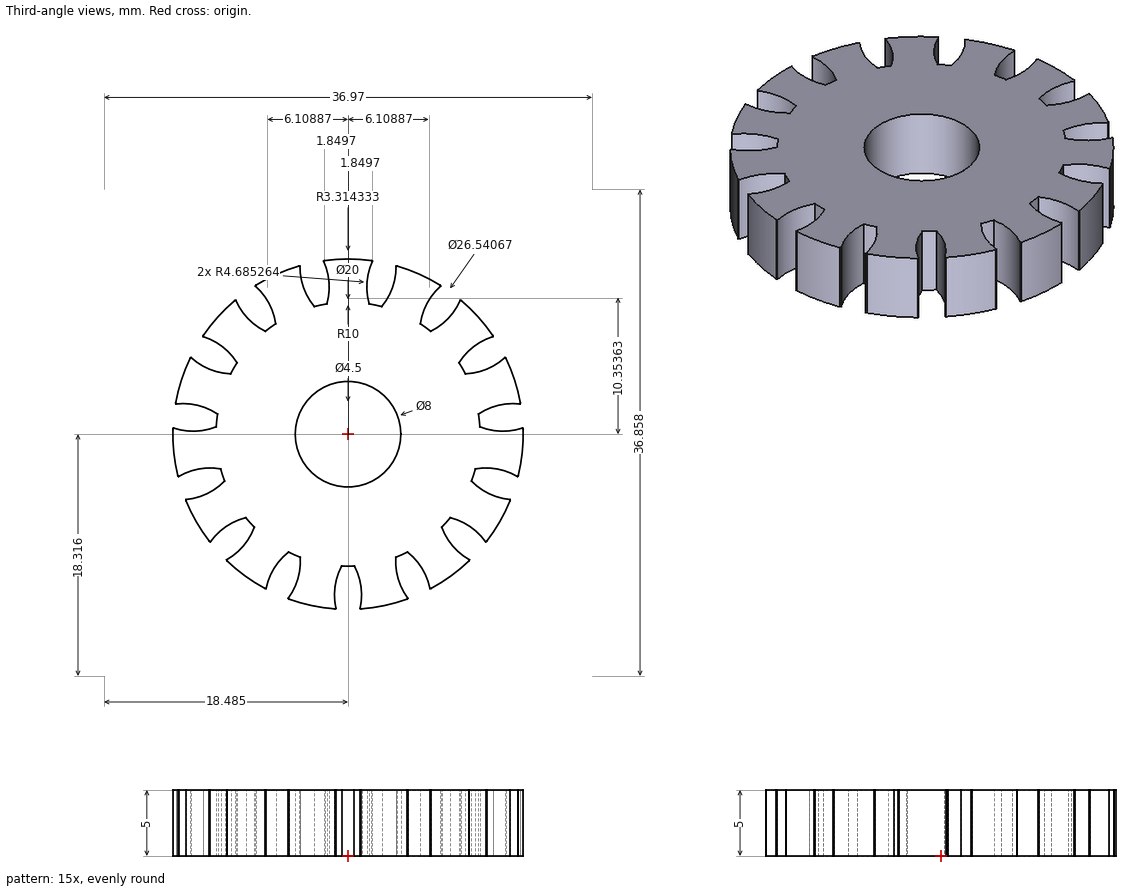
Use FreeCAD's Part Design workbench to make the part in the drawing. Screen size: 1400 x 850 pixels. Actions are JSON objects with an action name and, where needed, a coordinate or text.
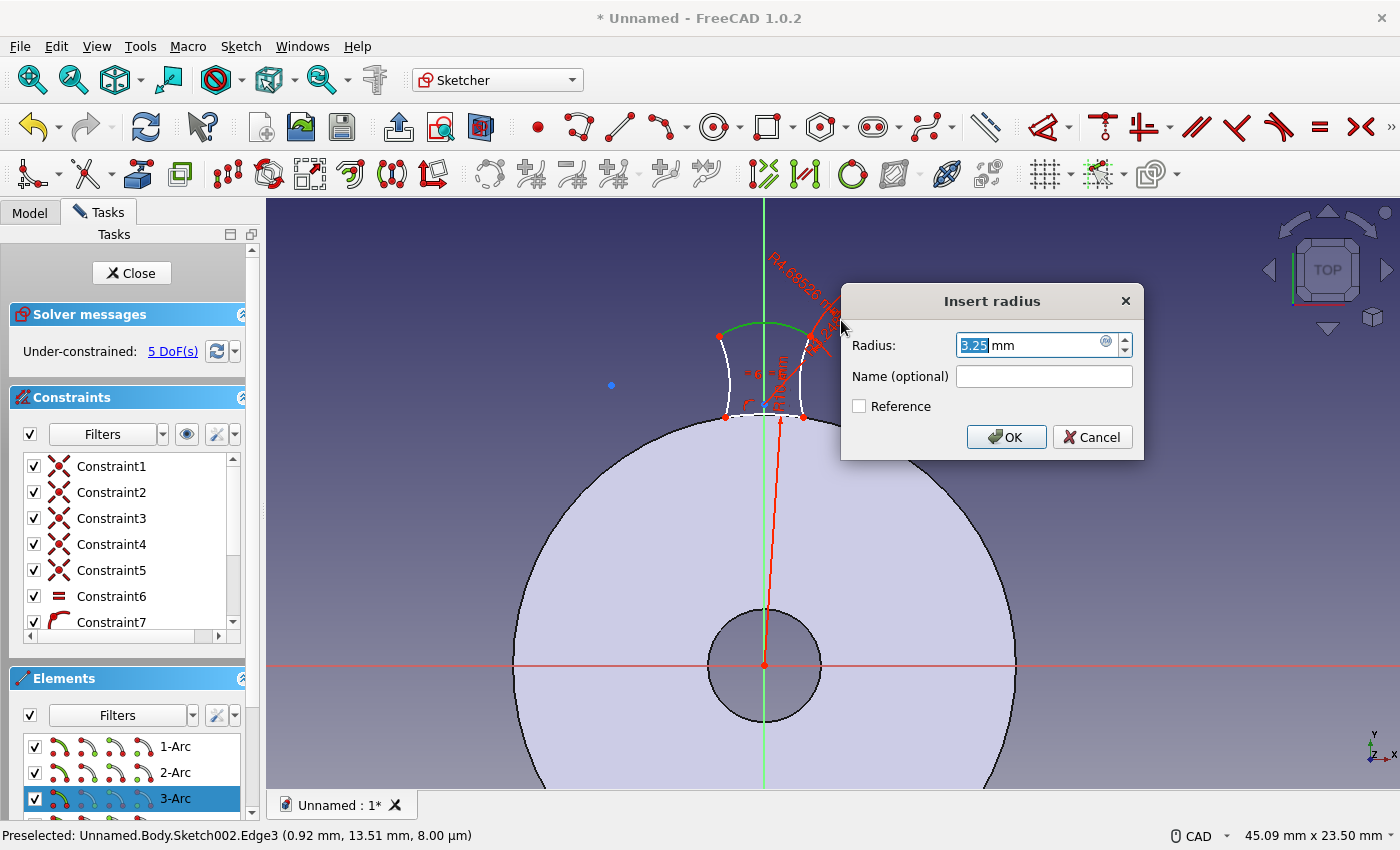
{"action": "type", "text": "3.314333"}
{"action": "key", "text": "Return"}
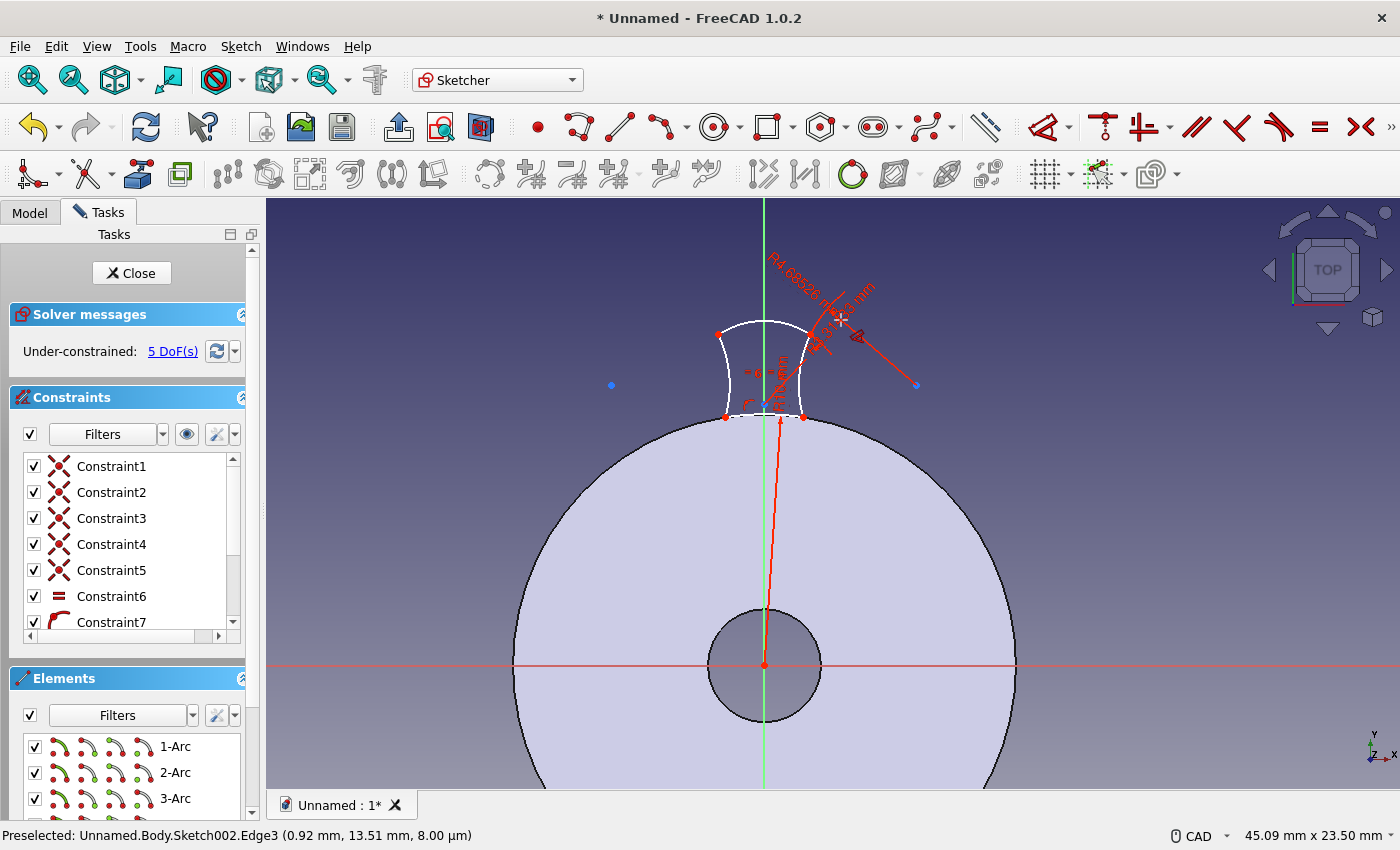
{"action": "left_click", "coordinate": [810, 335]}
{"action": "left_click", "coordinate": [787, 700]}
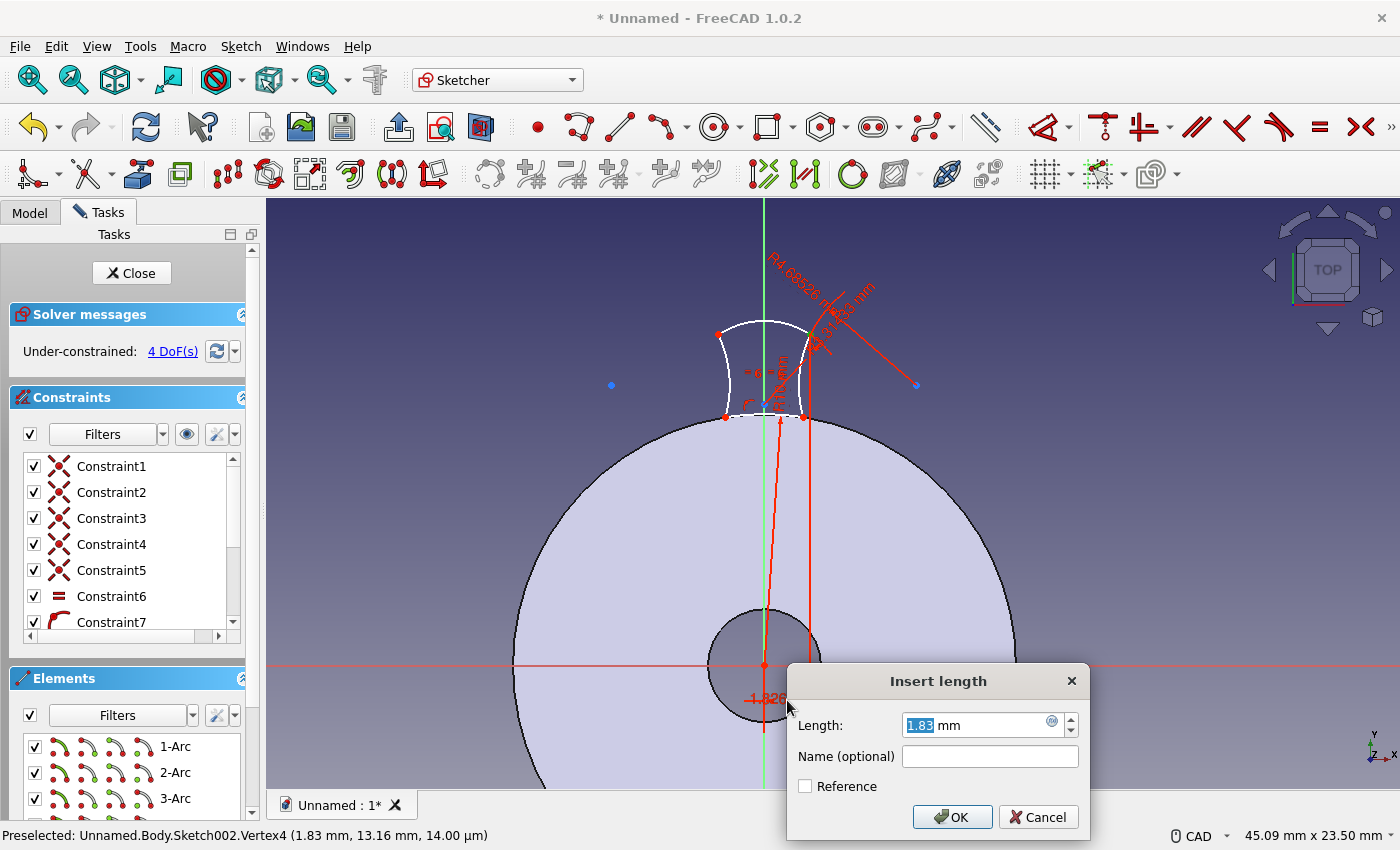
{"action": "type", "text": "1.8497"}
{"action": "key", "text": "Return"}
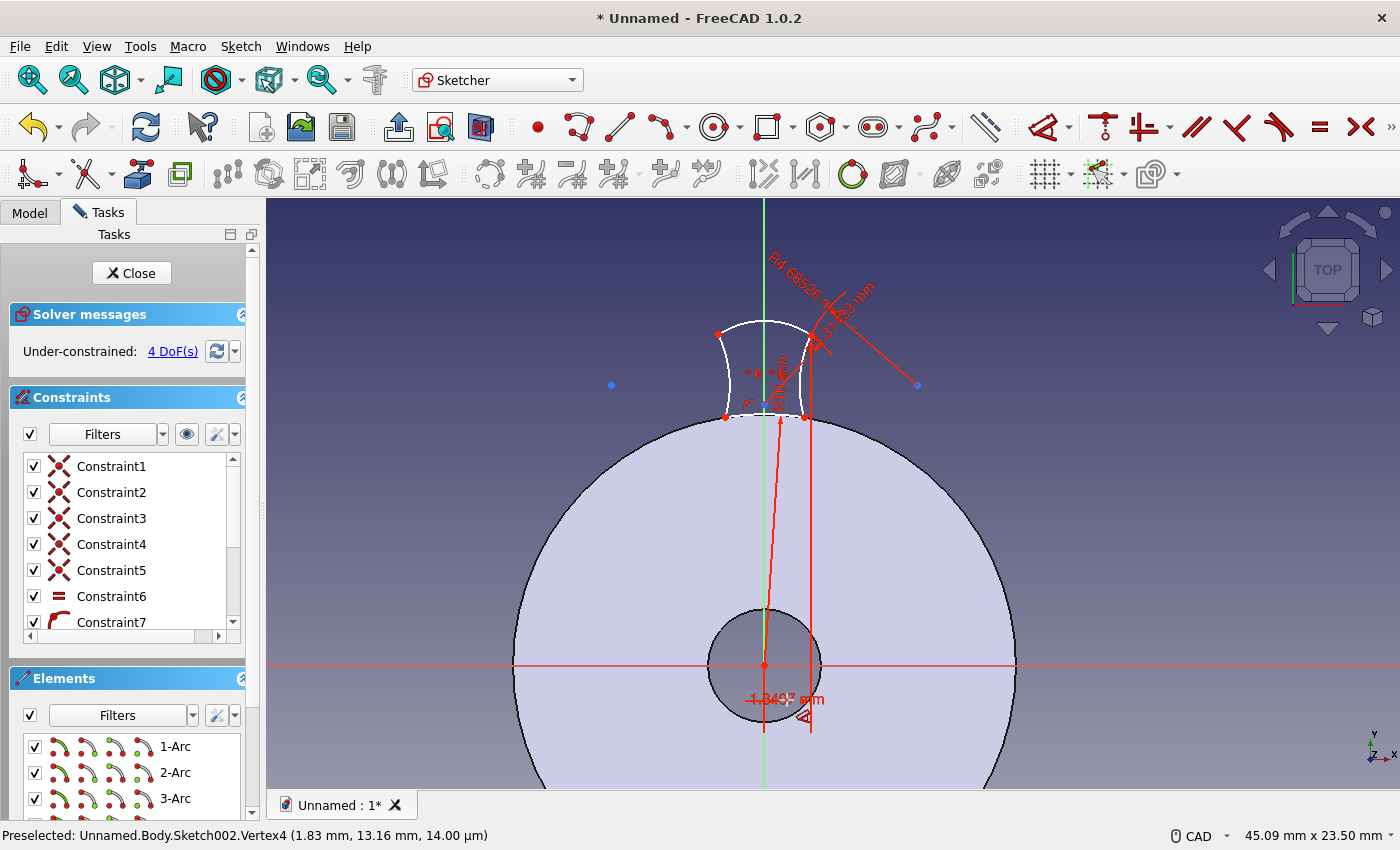
{"action": "left_click", "coordinate": [718, 335]}
{"action": "left_click", "coordinate": [731, 301]}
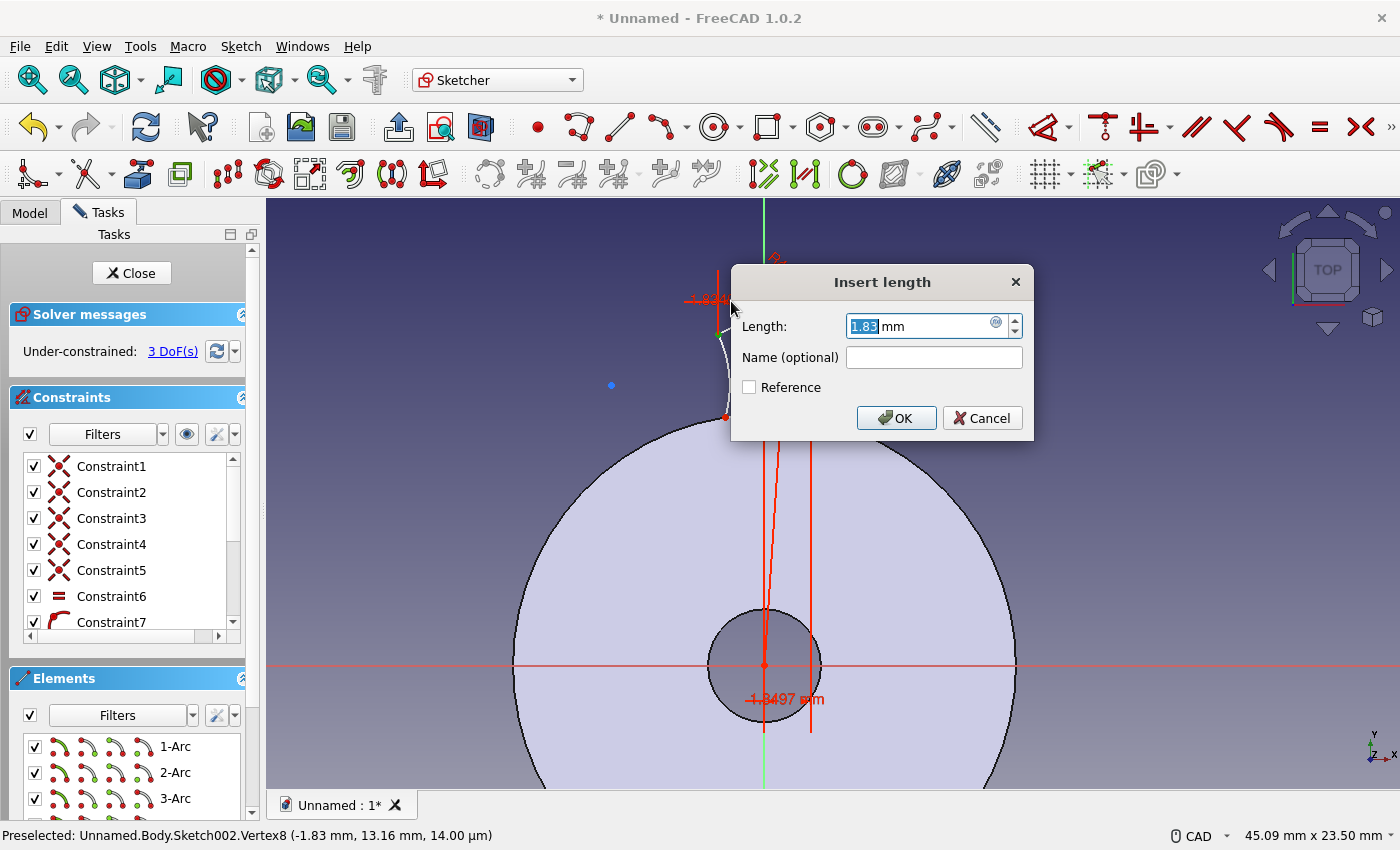
{"action": "type", "text": "1.8497"}
{"action": "key", "text": "Return"}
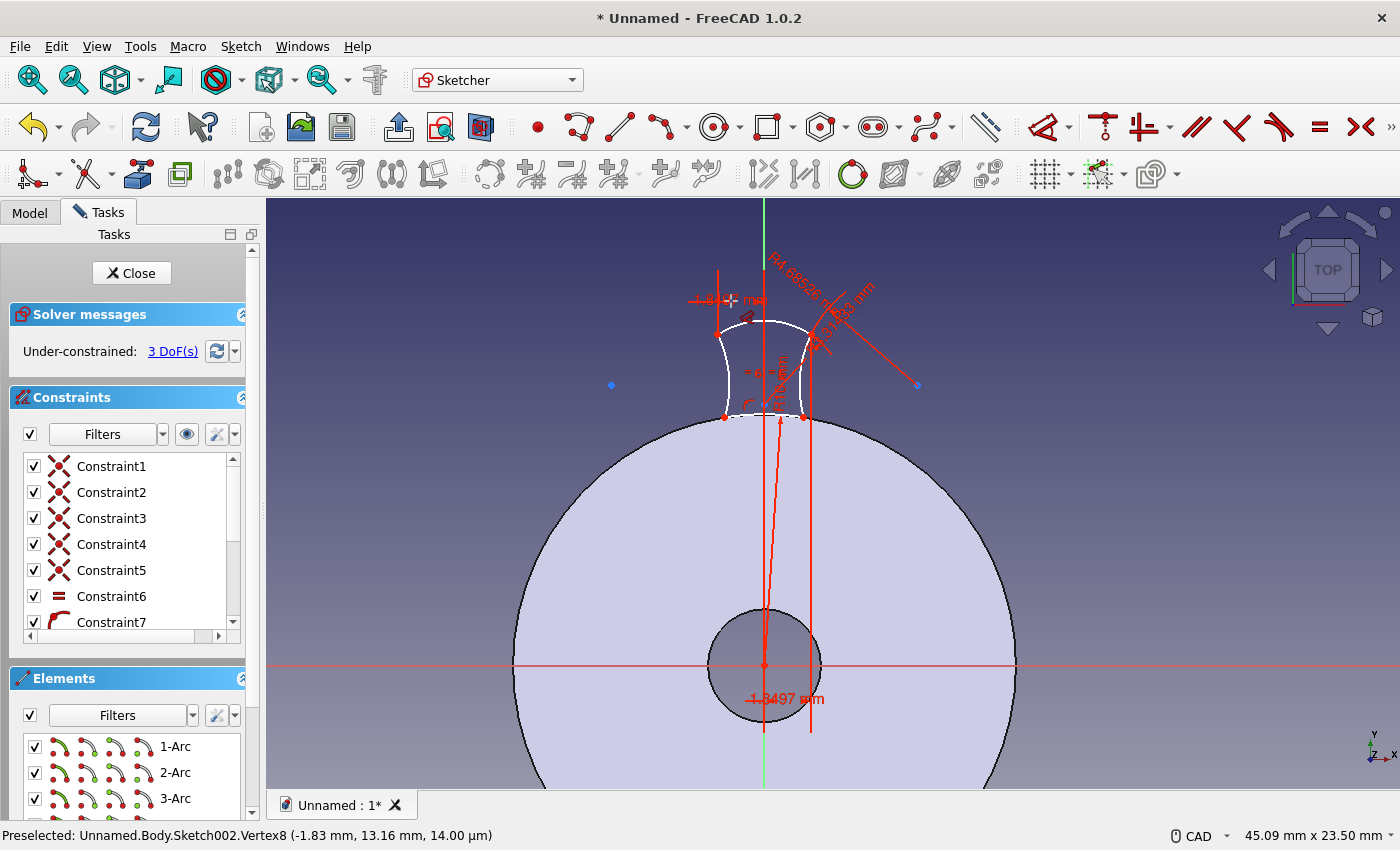
{"action": "left_click", "coordinate": [917, 385]}
{"action": "left_click", "coordinate": [876, 700]}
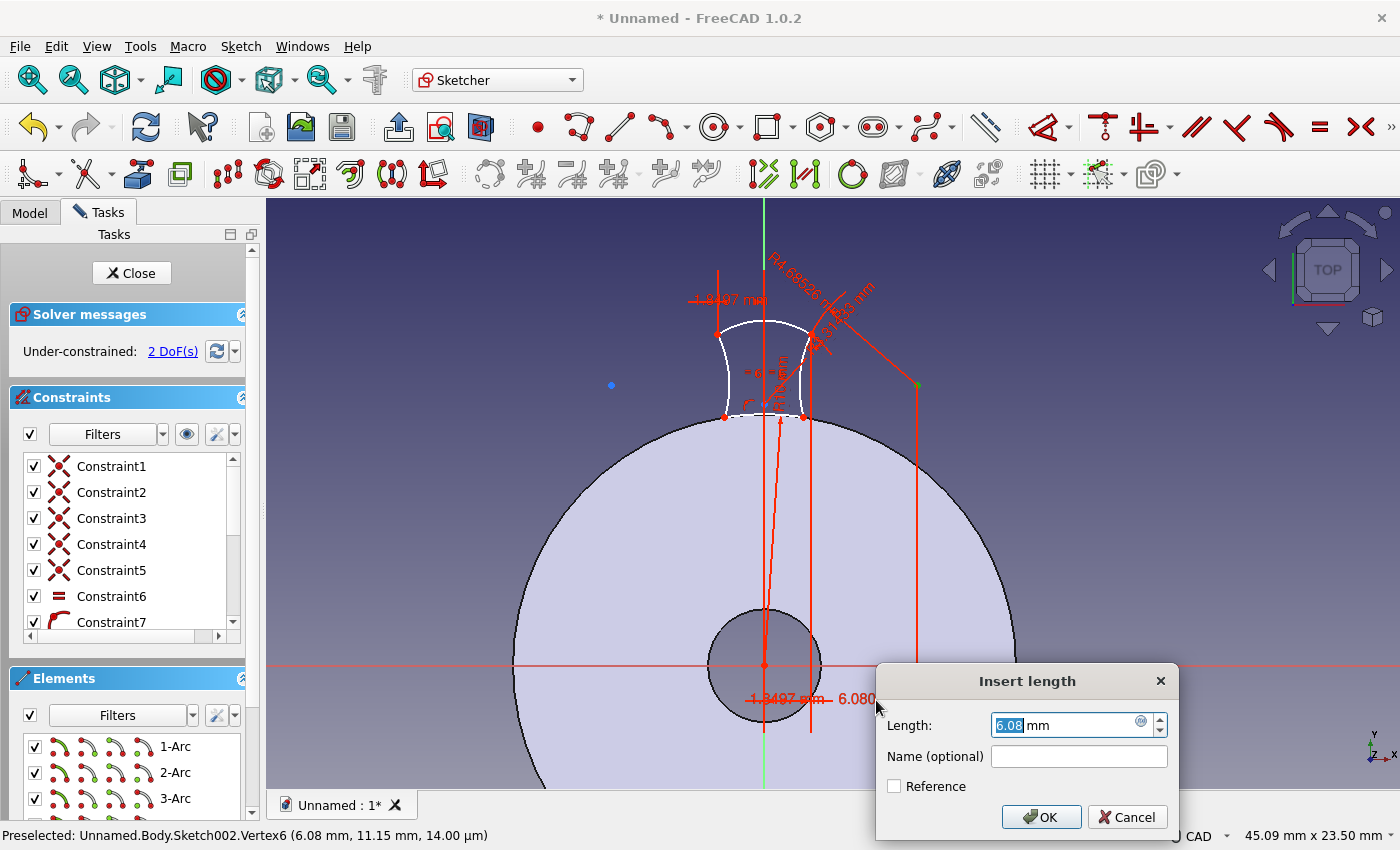
{"action": "type", "text": "6.10887"}
{"action": "key", "text": "Return"}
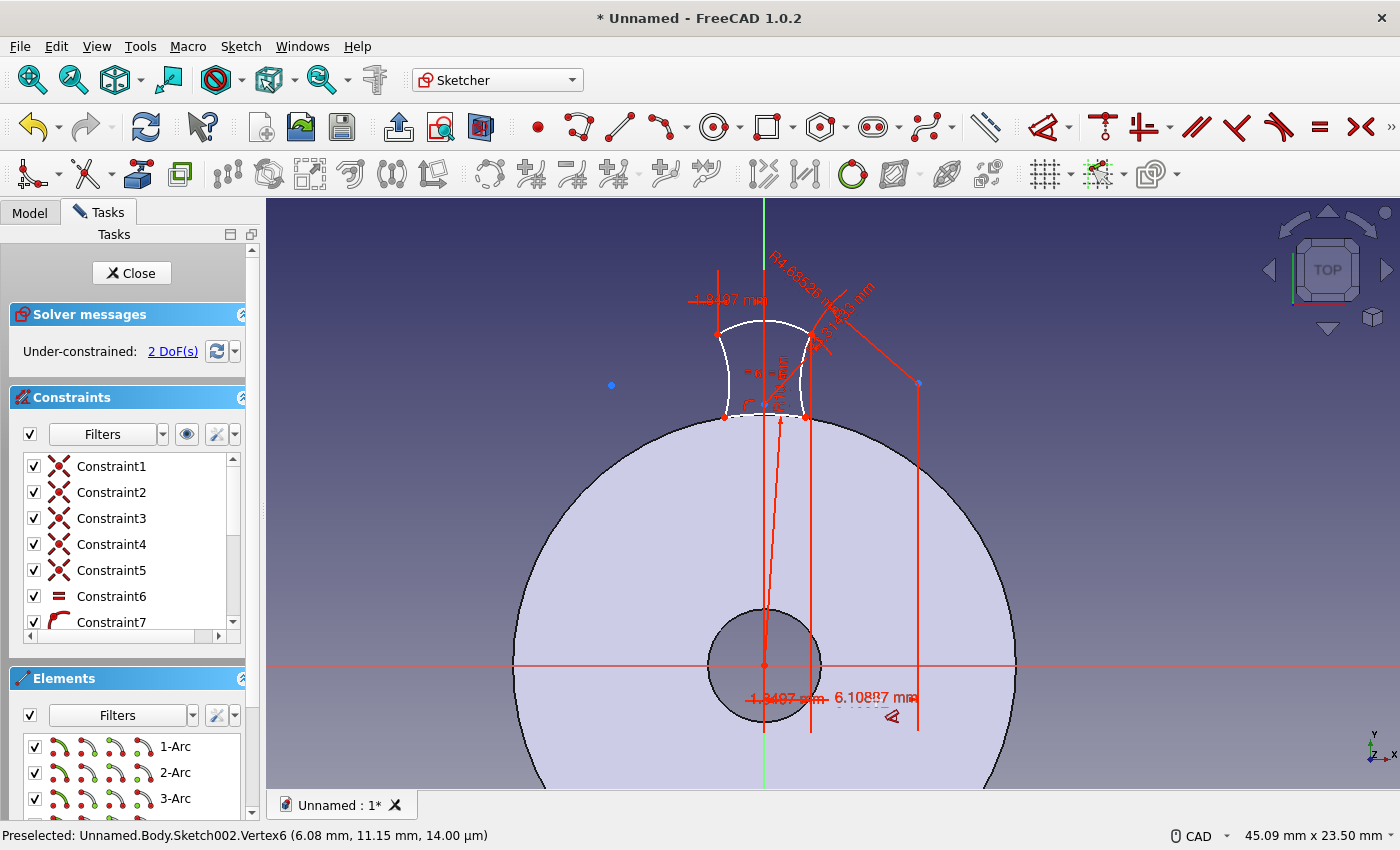
{"action": "left_click", "coordinate": [612, 385]}
{"action": "left_click", "coordinate": [688, 700]}